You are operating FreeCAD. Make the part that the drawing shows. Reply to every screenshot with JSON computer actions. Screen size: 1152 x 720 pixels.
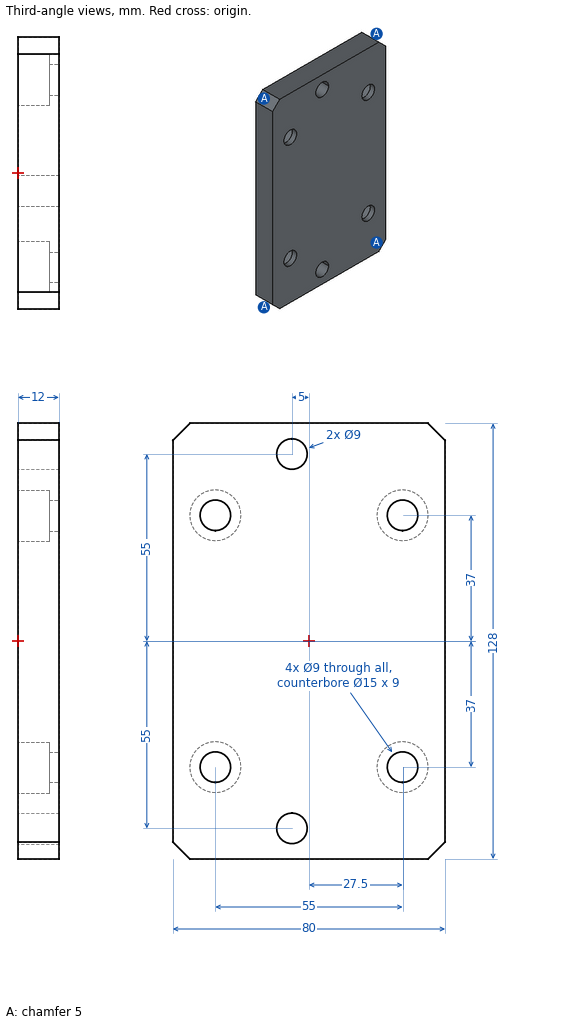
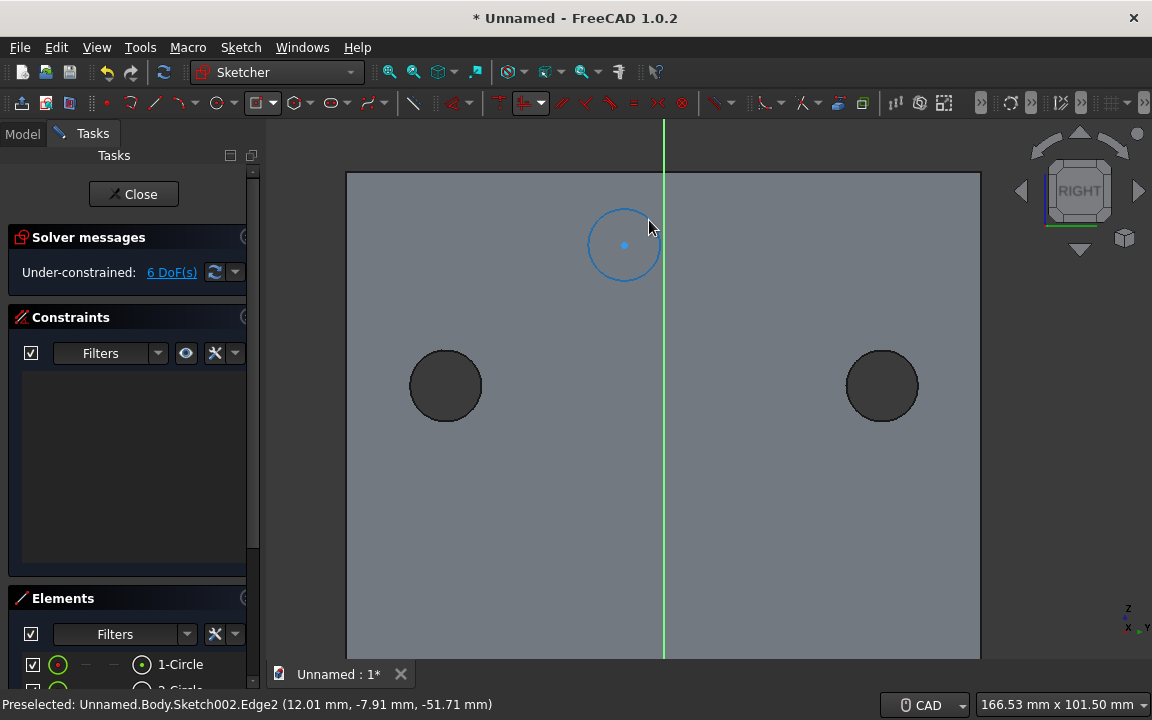
{"action": "left_click", "coordinate": [650, 220]}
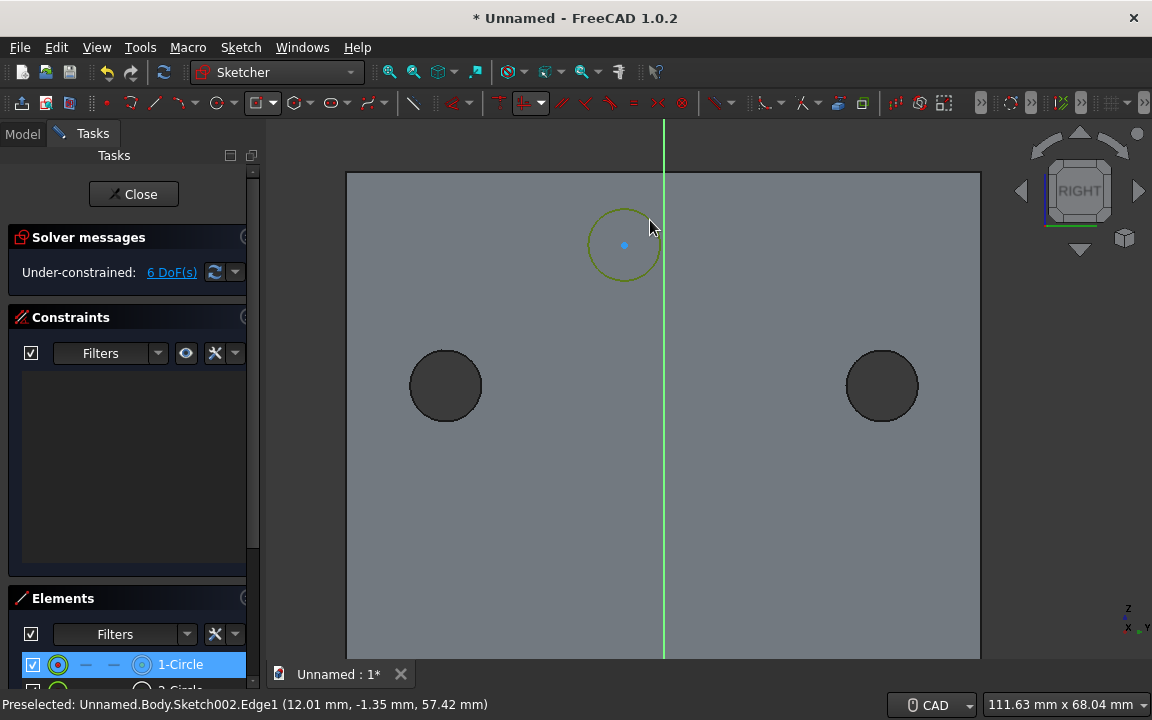
{"action": "scroll", "coordinate": [649, 220], "scroll_direction": "down", "scroll_amount": 5}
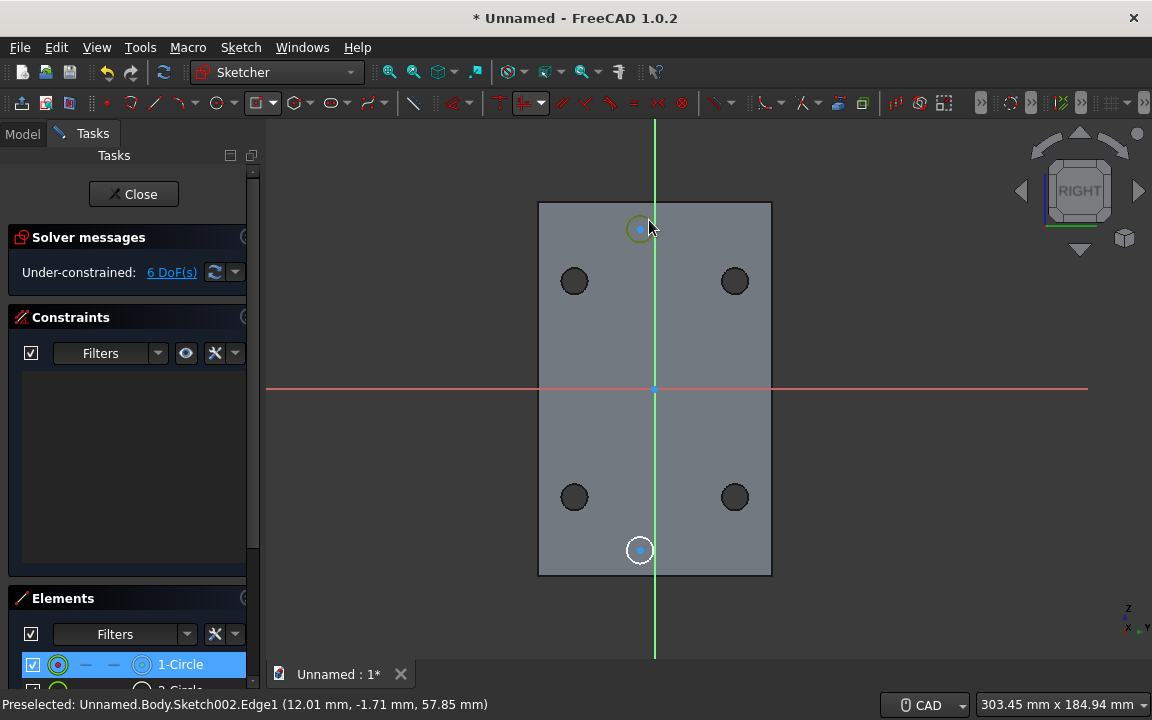
{"action": "scroll", "coordinate": [649, 541], "scroll_direction": "up", "scroll_amount": 5}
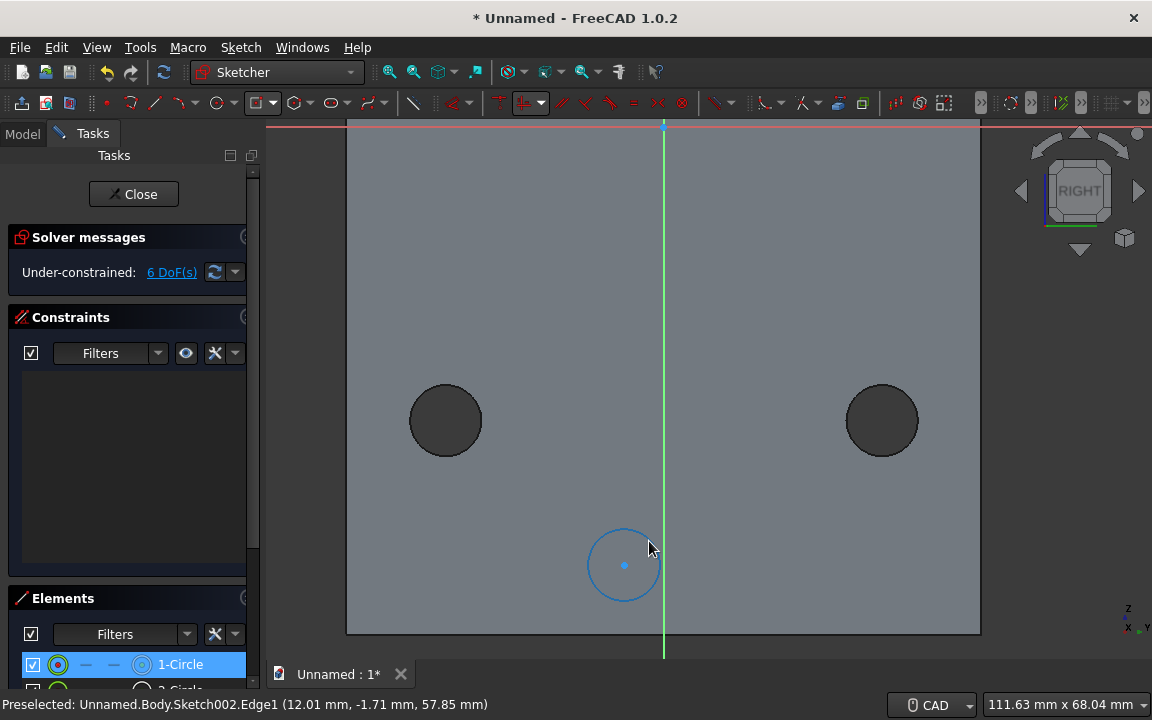
{"action": "left_click", "coordinate": [649, 540]}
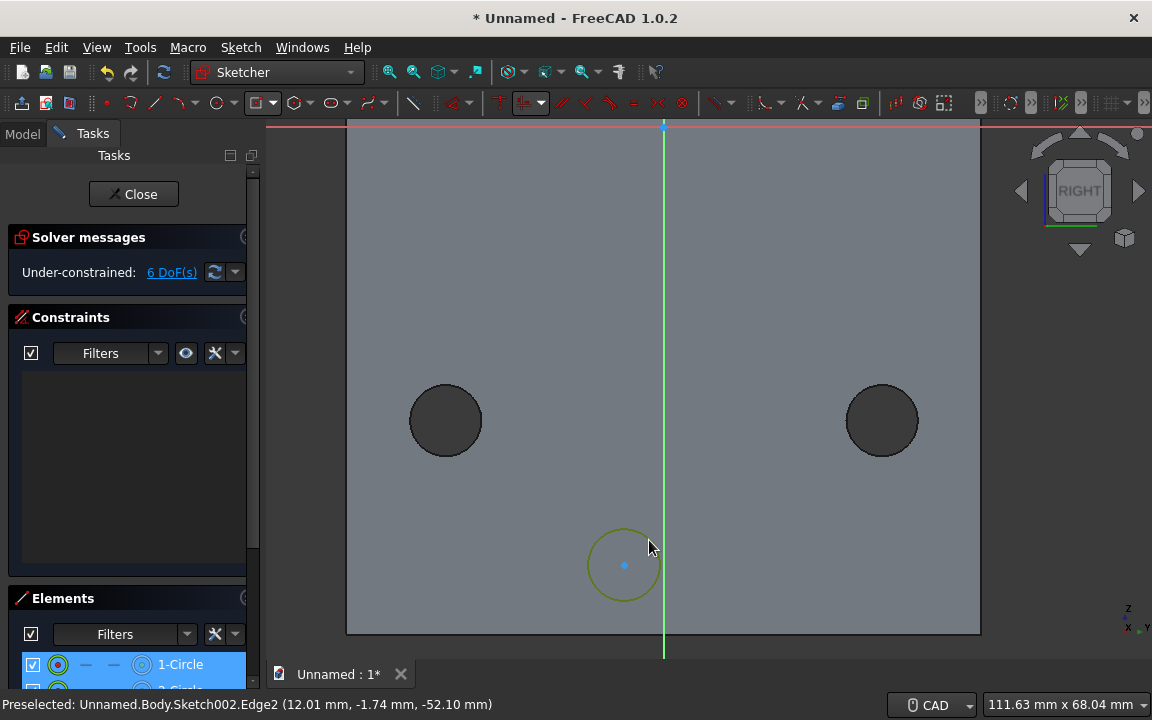
{"action": "left_click", "coordinate": [634, 104]}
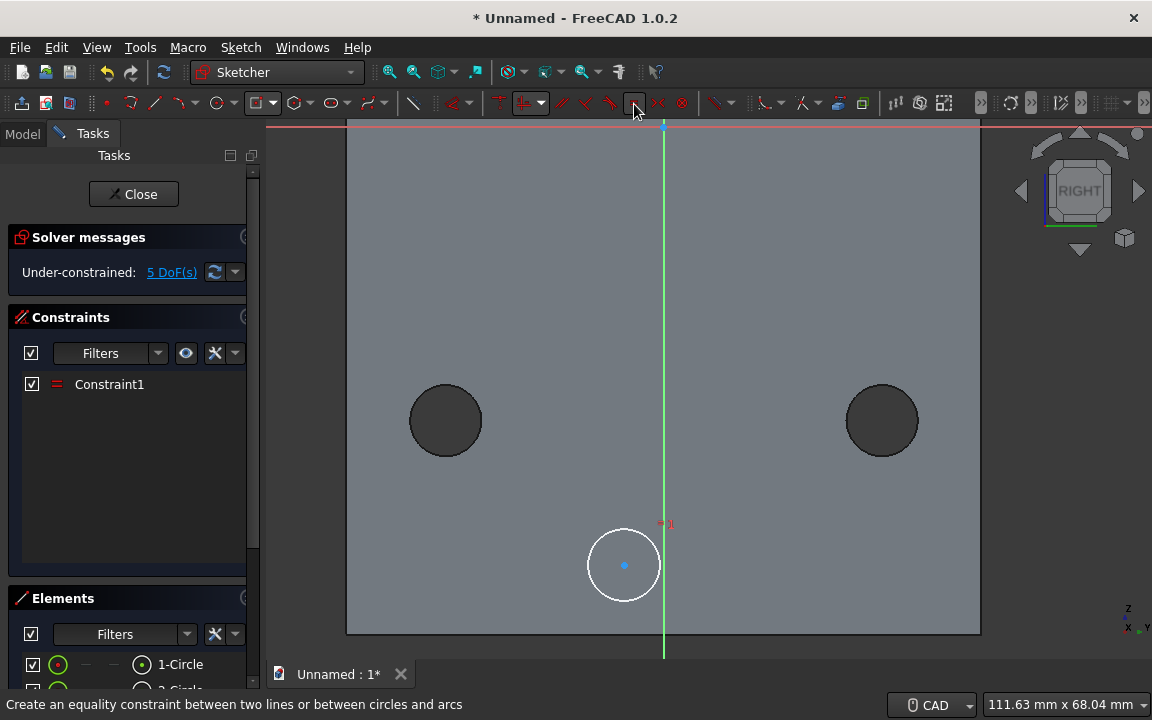
{"action": "scroll", "coordinate": [649, 541], "scroll_direction": "down", "scroll_amount": 5}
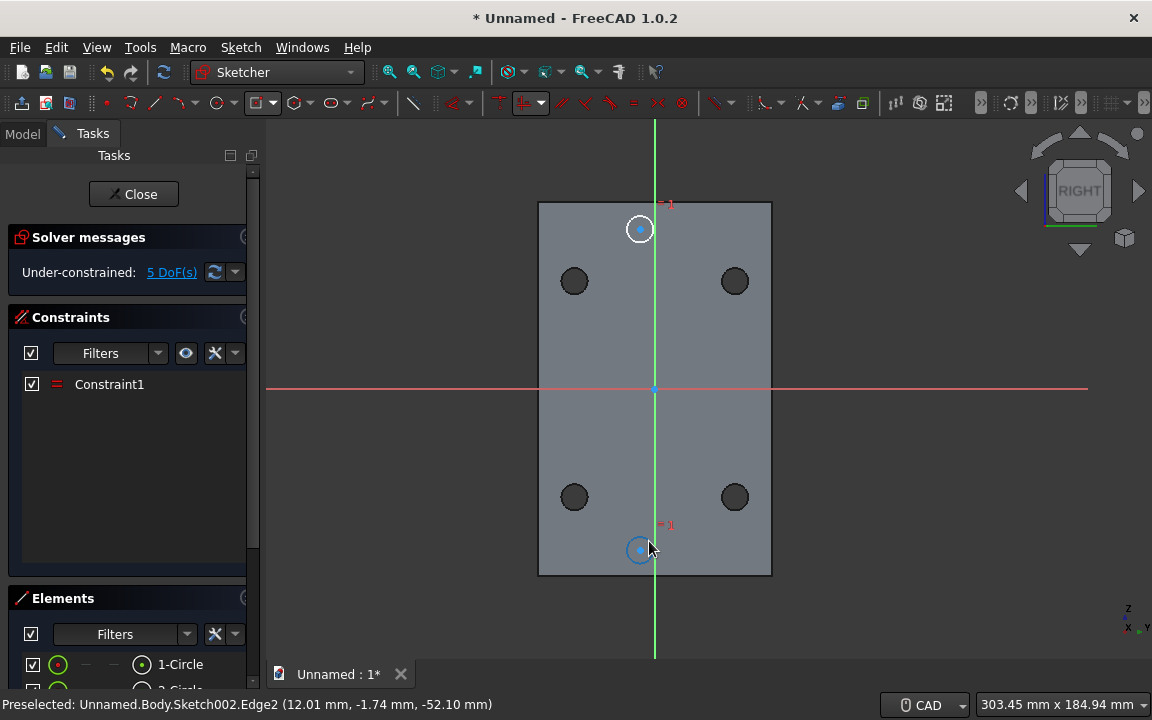
{"action": "left_click", "coordinate": [640, 229]}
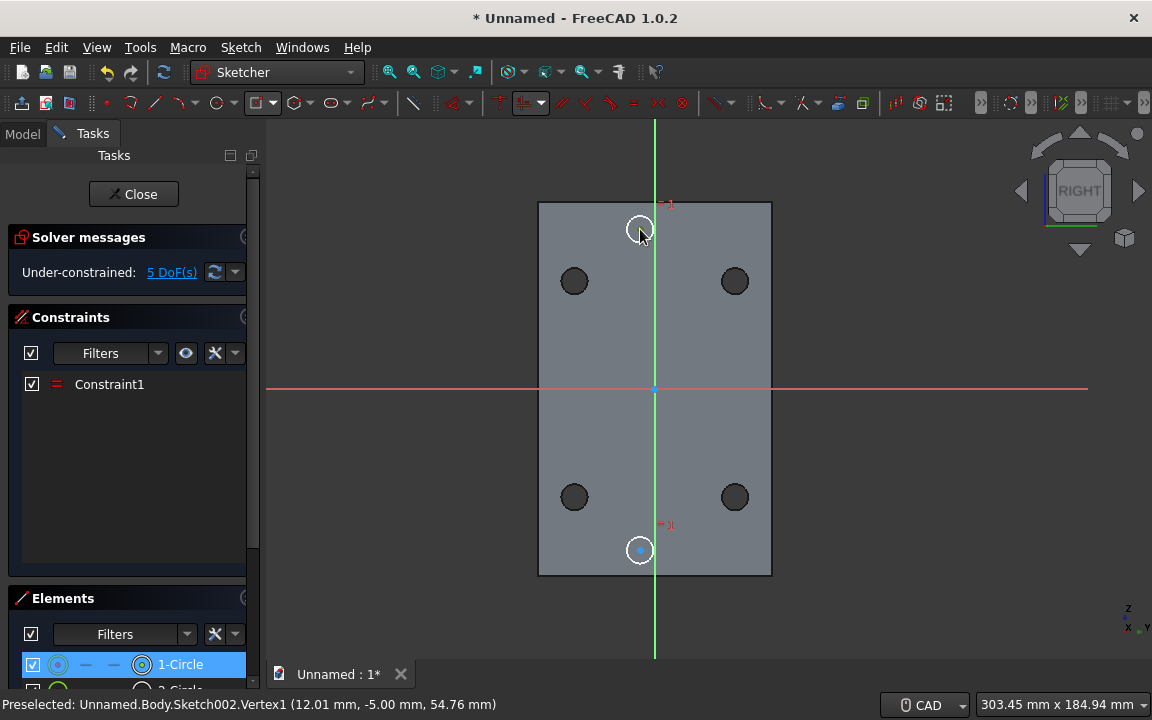
{"action": "left_click", "coordinate": [640, 550]}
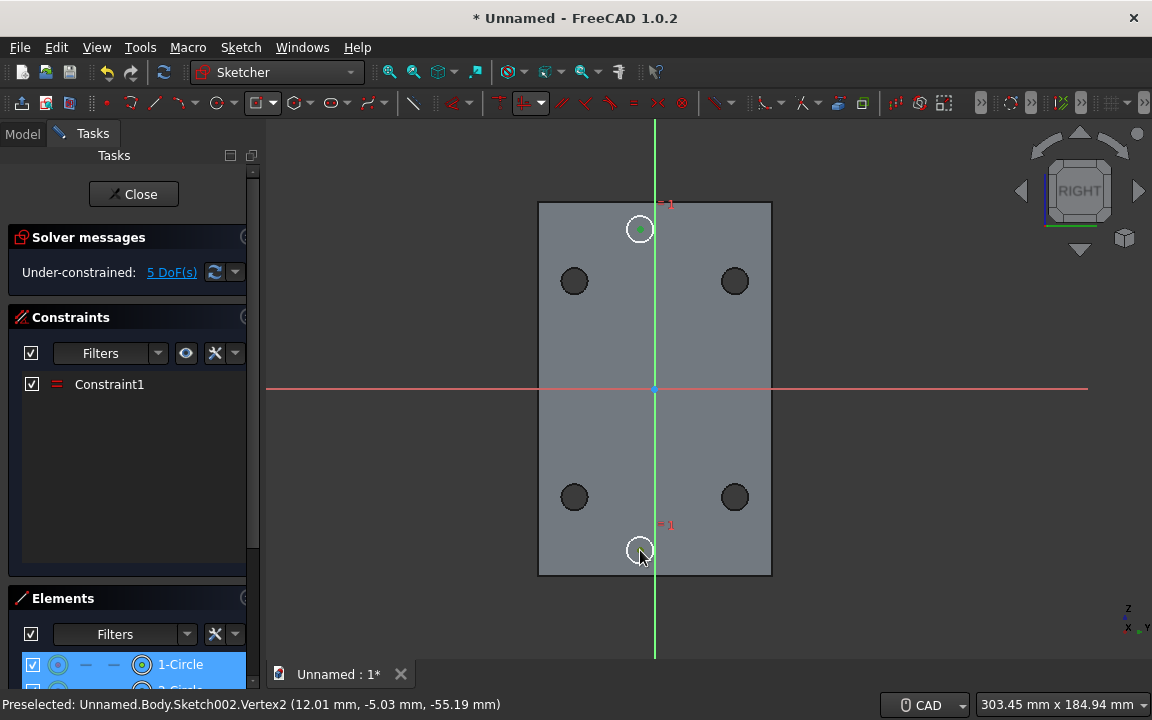
{"action": "key", "text": "v"}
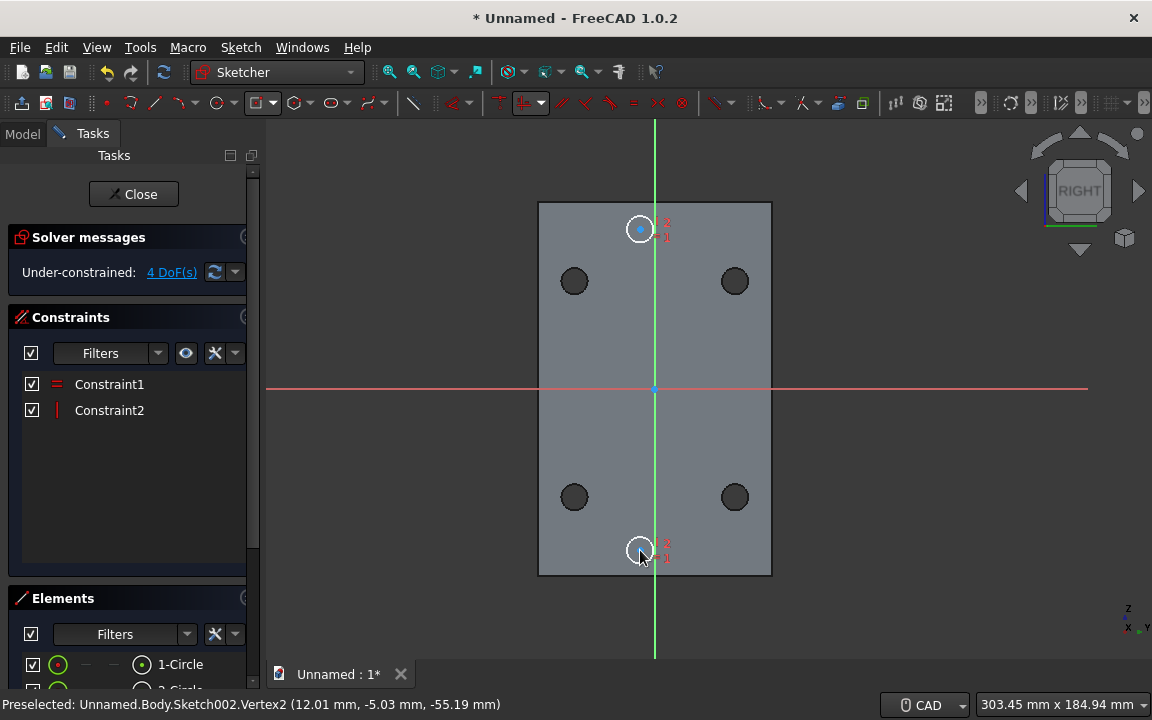
{"action": "left_click", "coordinate": [452, 104]}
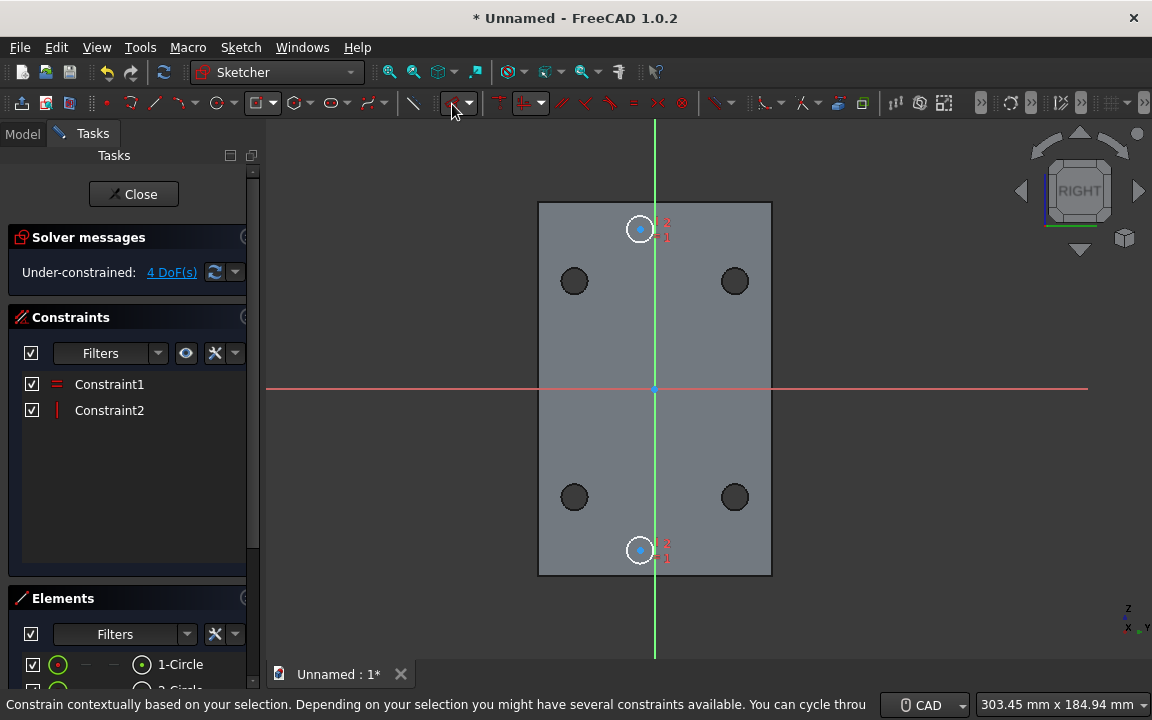
{"action": "scroll", "coordinate": [631, 220], "scroll_direction": "up", "scroll_amount": 3}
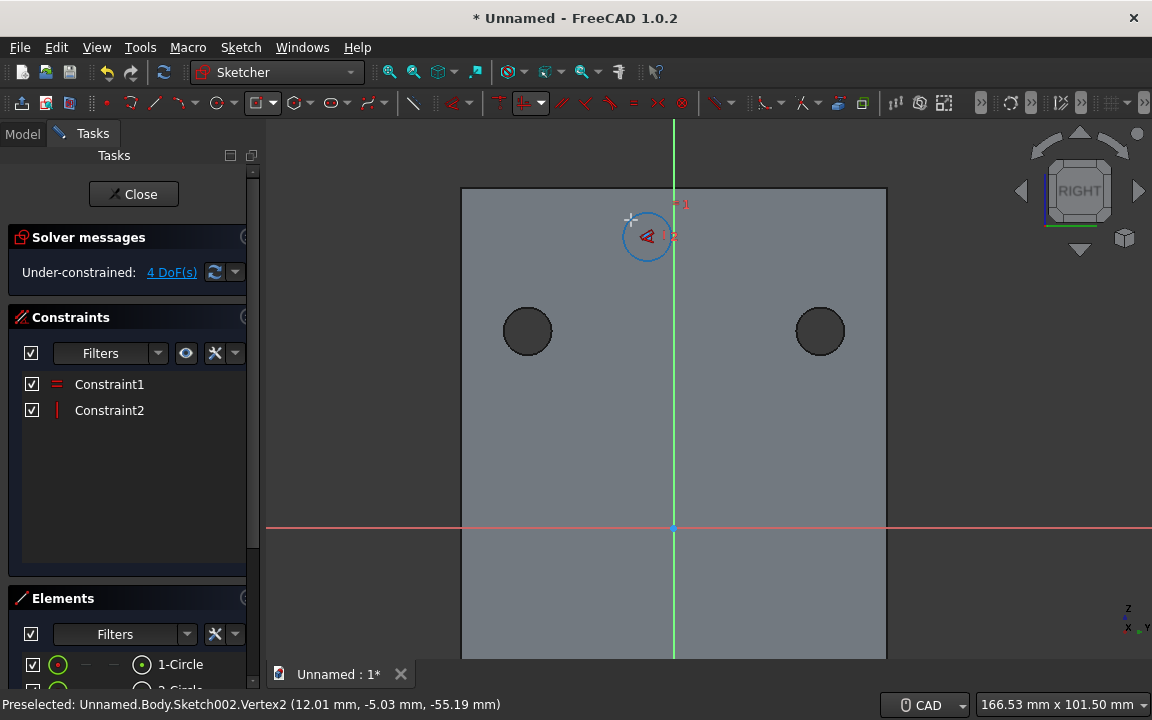
{"action": "left_click", "coordinate": [630, 220]}
{"action": "left_click", "coordinate": [607, 198]}